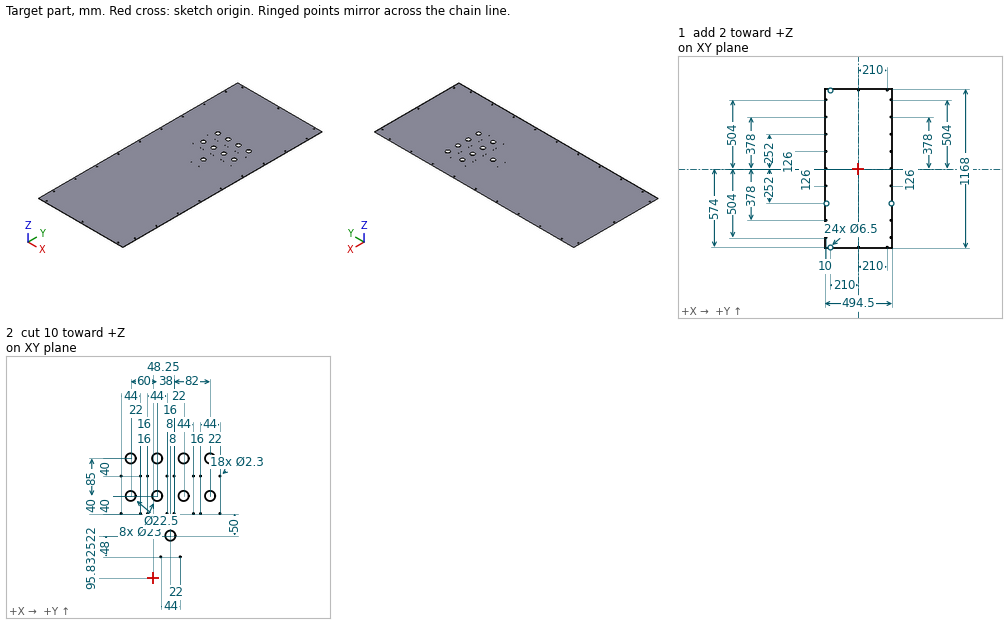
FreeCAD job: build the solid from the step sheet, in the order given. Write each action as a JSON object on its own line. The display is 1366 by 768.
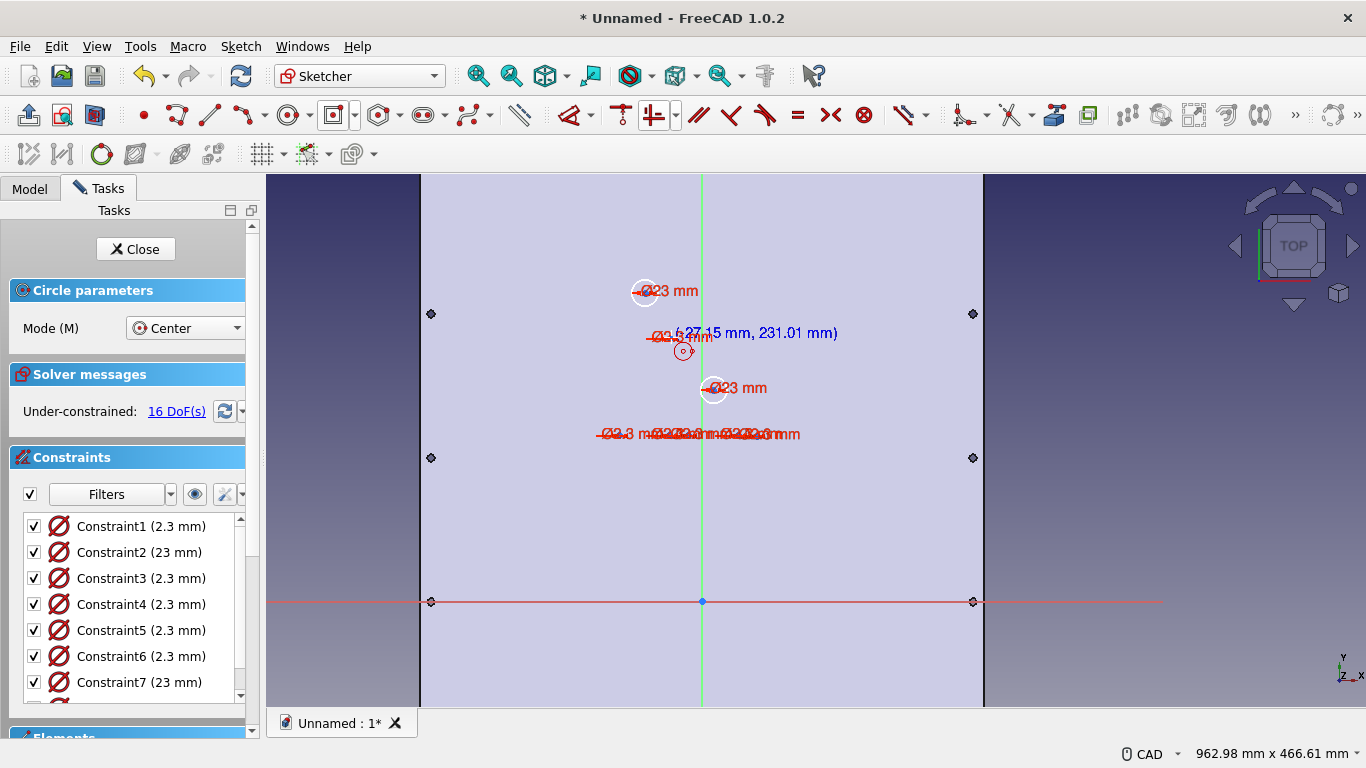
{"action": "scroll", "coordinate": [620, 338], "scroll_direction": "up", "scroll_amount": 15}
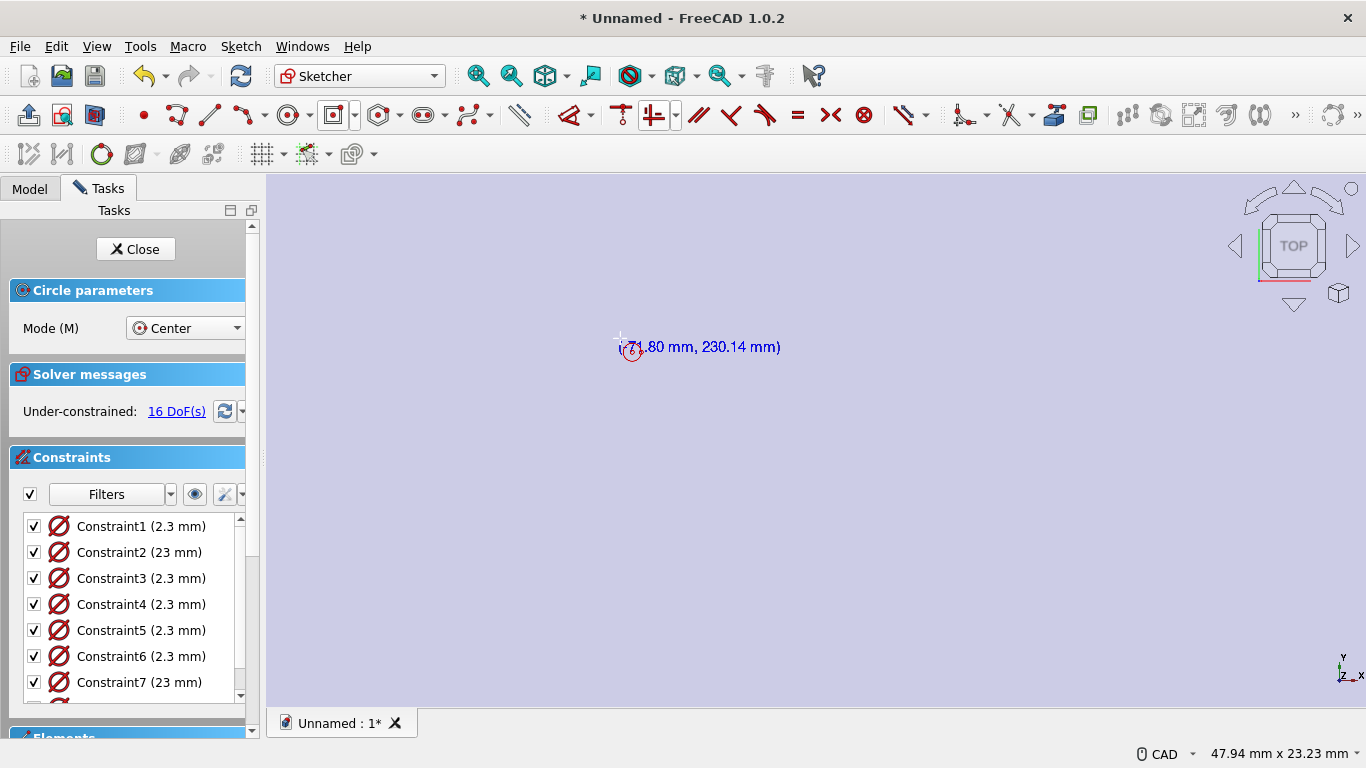
{"action": "scroll", "coordinate": [620, 338], "scroll_direction": "down", "scroll_amount": 15}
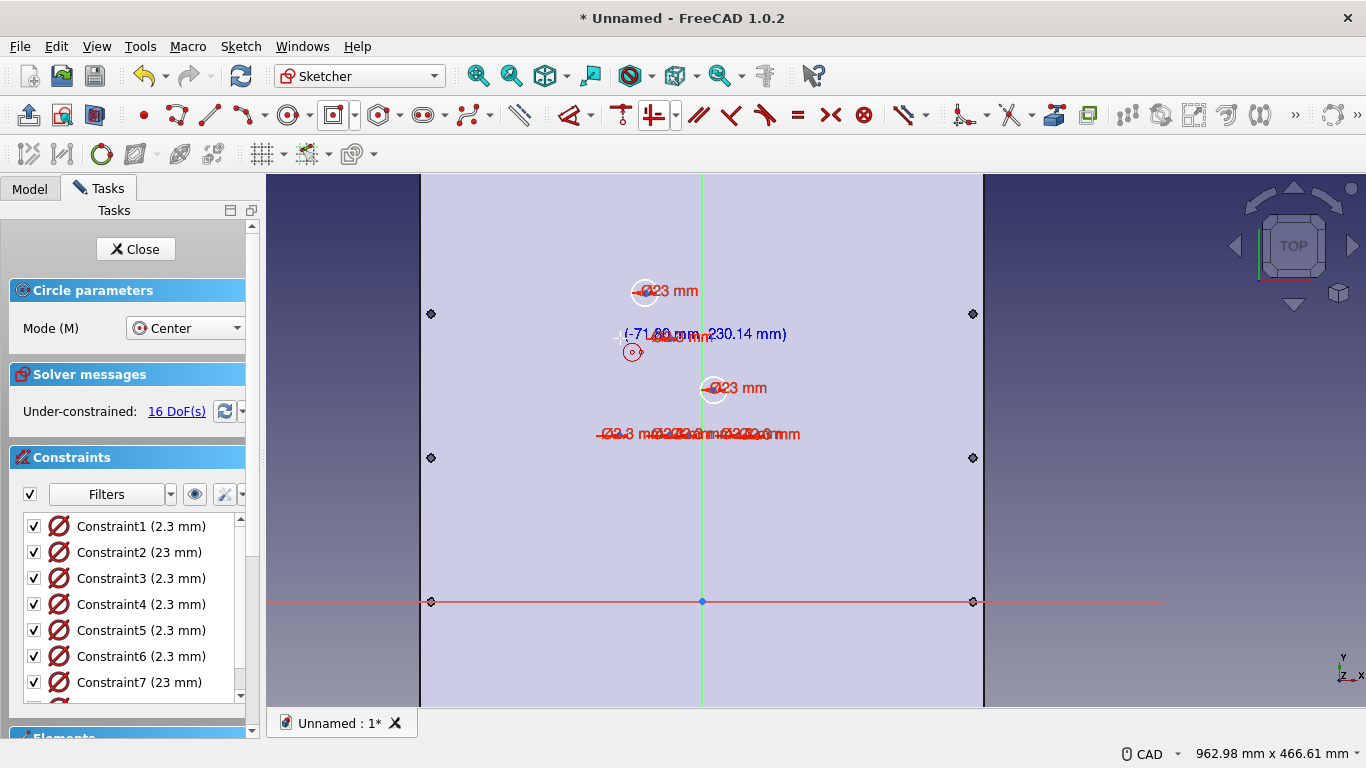
{"action": "left_click", "coordinate": [620, 338]}
{"action": "mouse_move", "coordinate": [621, 337]}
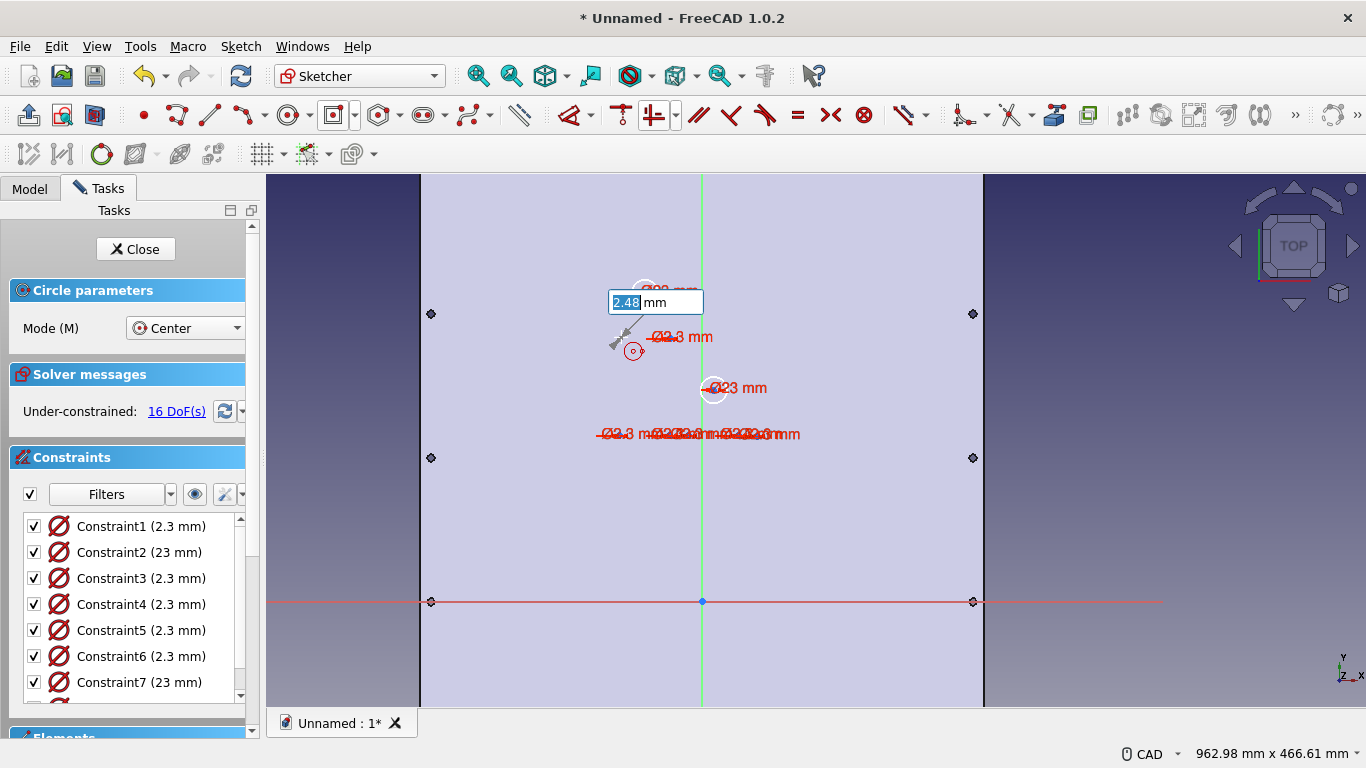
{"action": "type", "text": "2.3"}
{"action": "key", "text": "Return"}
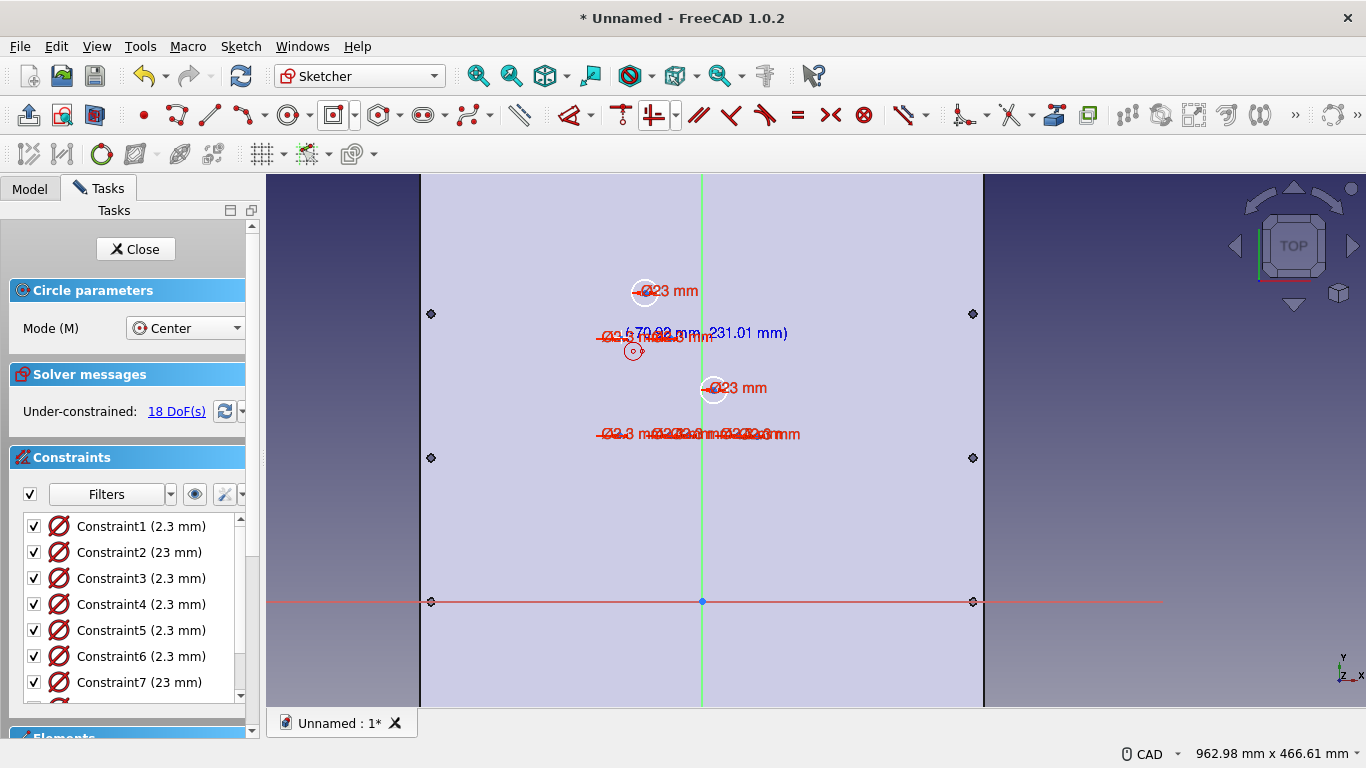
{"action": "scroll", "coordinate": [851, 390], "scroll_direction": "up", "scroll_amount": 3}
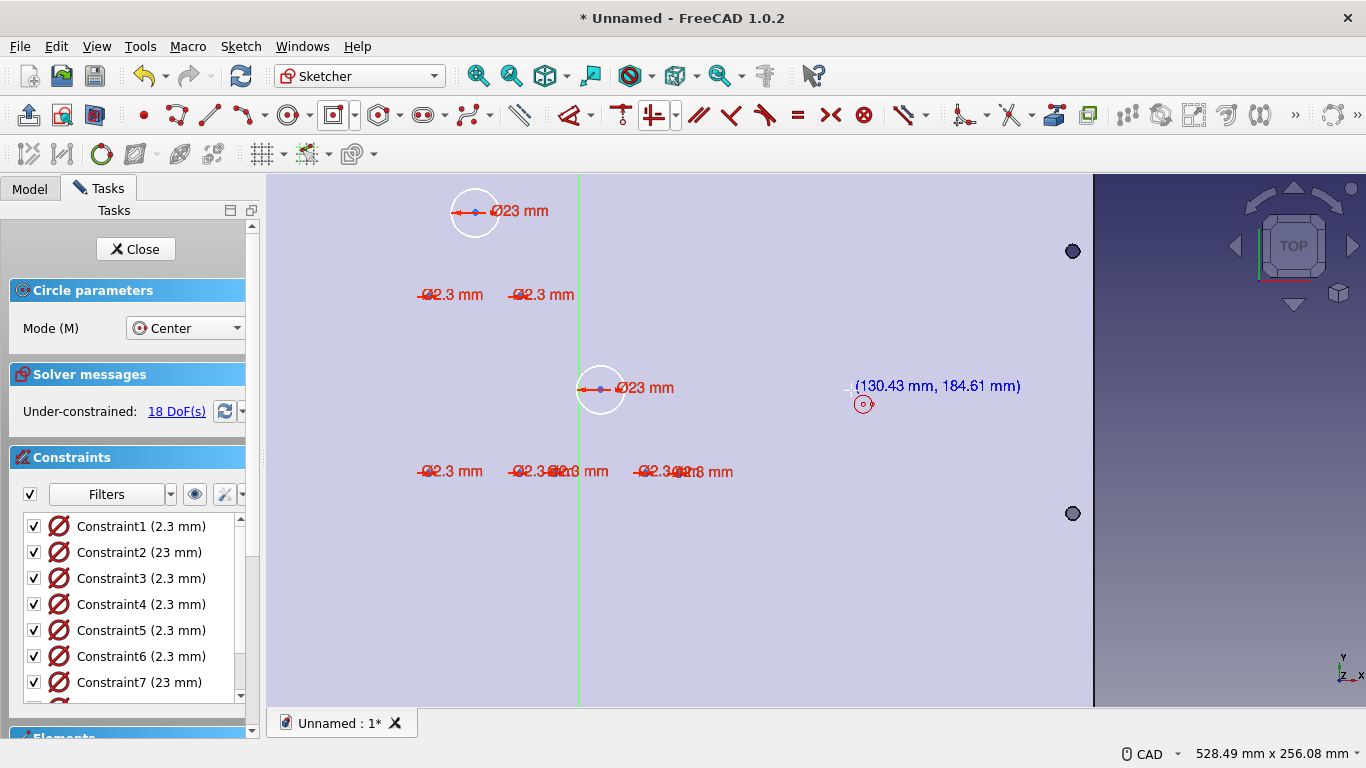
{"action": "left_click", "coordinate": [850, 389]}
{"action": "mouse_move", "coordinate": [867, 372]}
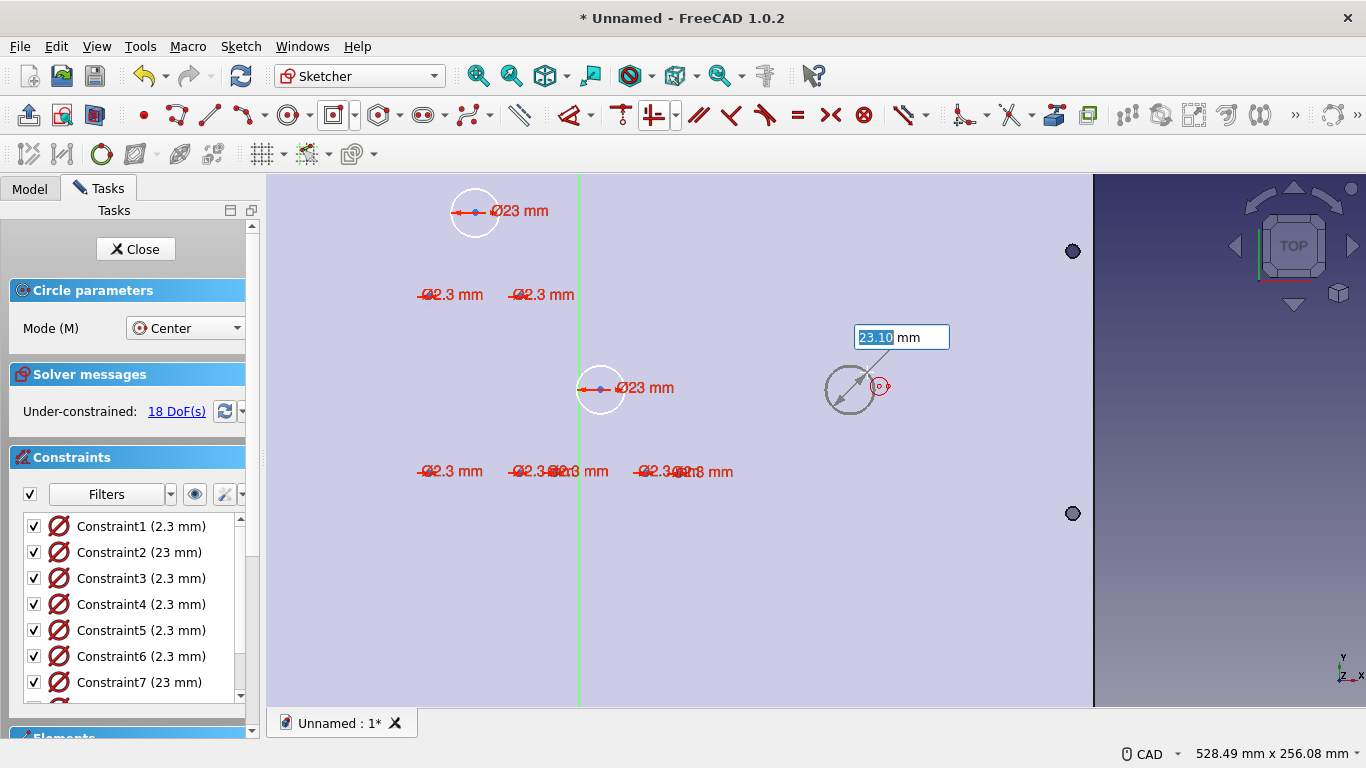
{"action": "type", "text": "23"}
{"action": "key", "text": "Return"}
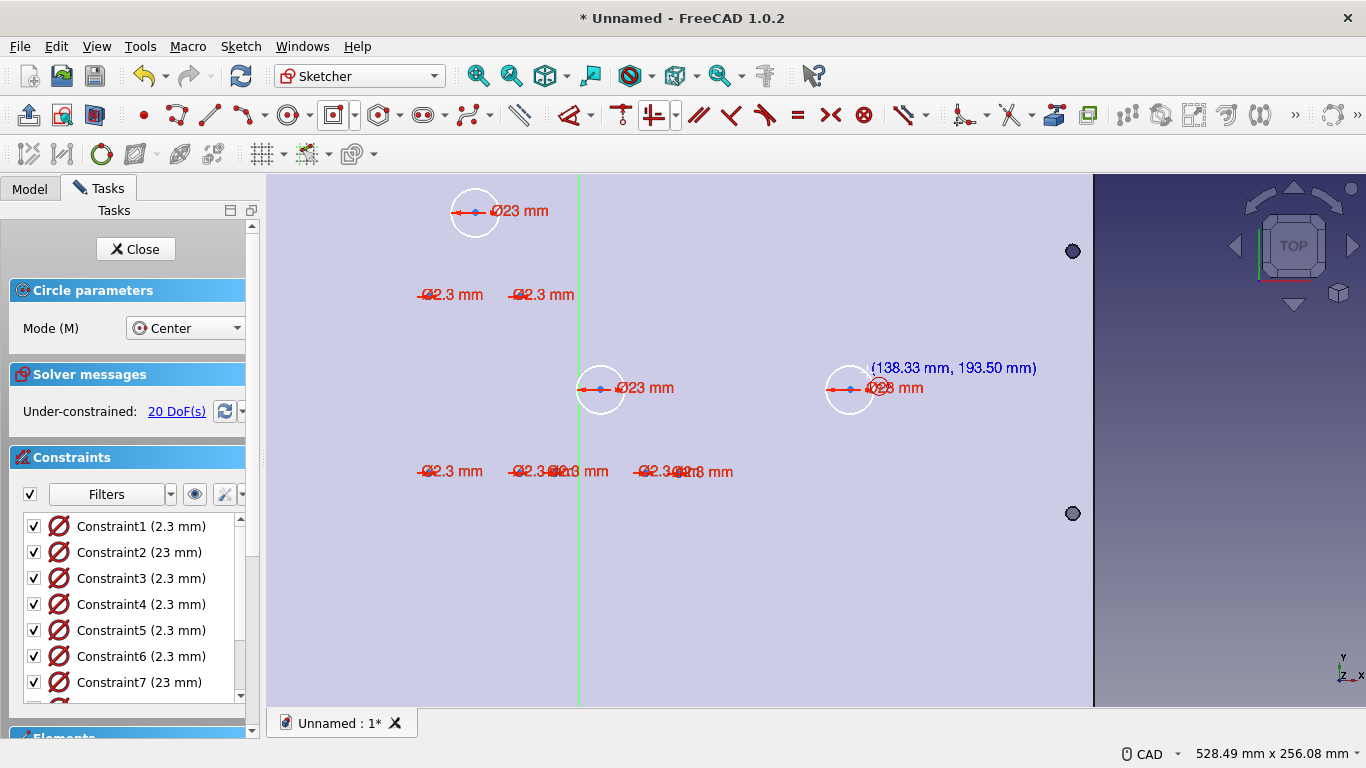
{"action": "scroll", "coordinate": [896, 472], "scroll_direction": "up", "scroll_amount": 12}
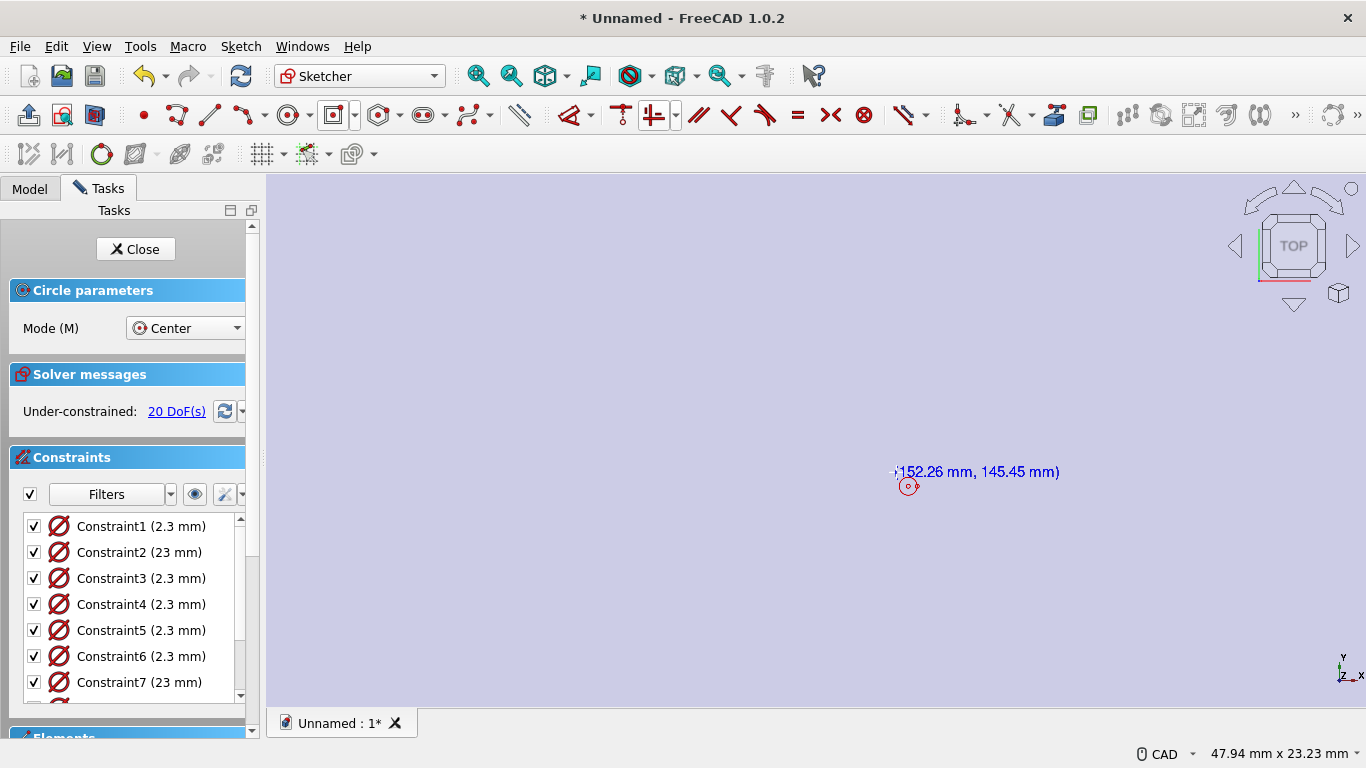
{"action": "scroll", "coordinate": [875, 433], "scroll_direction": "down", "scroll_amount": 15}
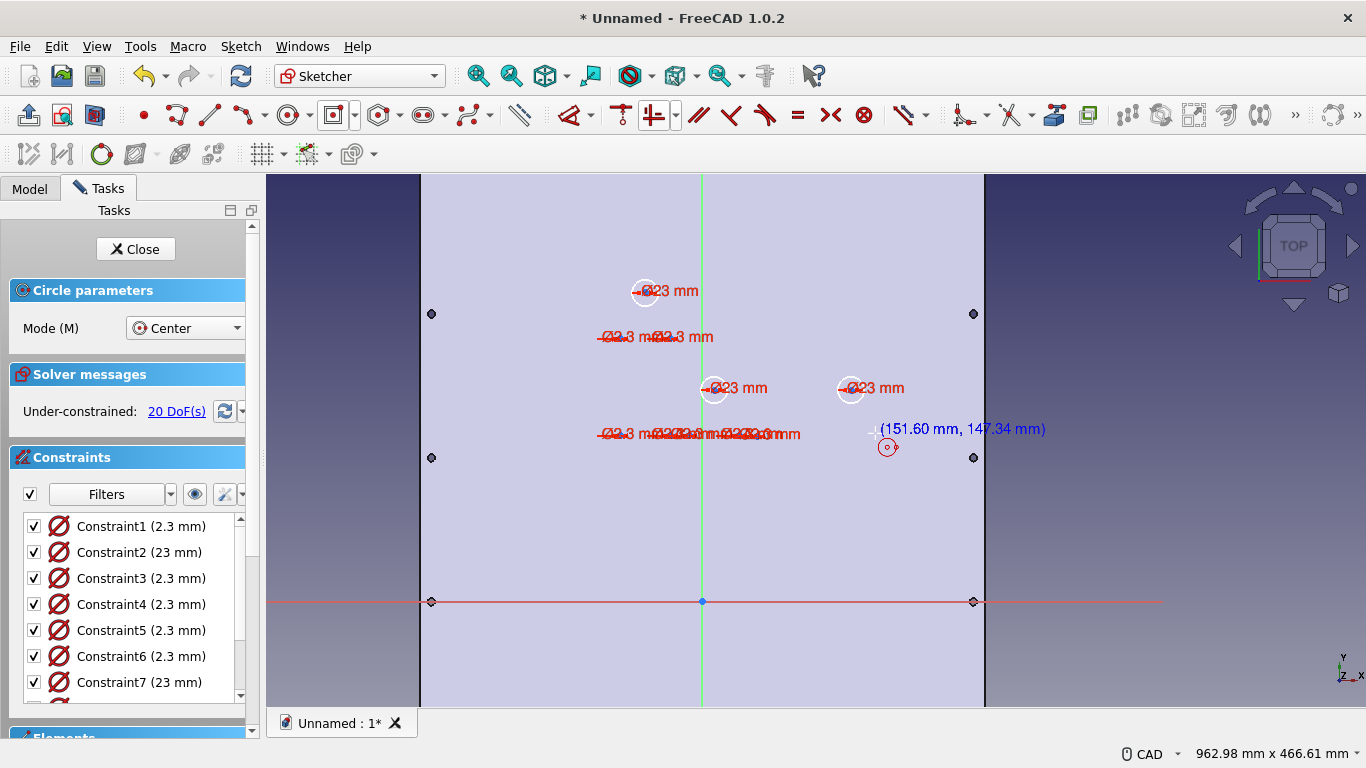
{"action": "left_click", "coordinate": [876, 435]}
{"action": "mouse_move", "coordinate": [877, 434]}